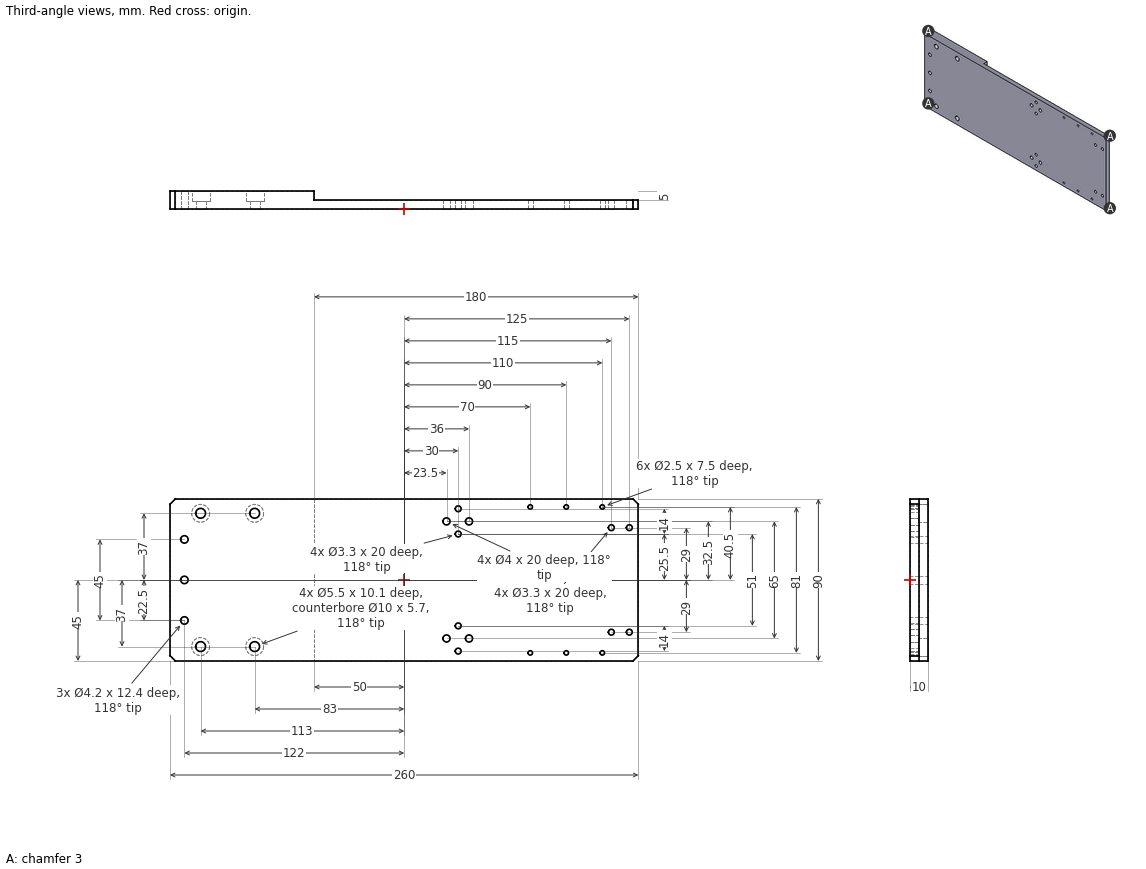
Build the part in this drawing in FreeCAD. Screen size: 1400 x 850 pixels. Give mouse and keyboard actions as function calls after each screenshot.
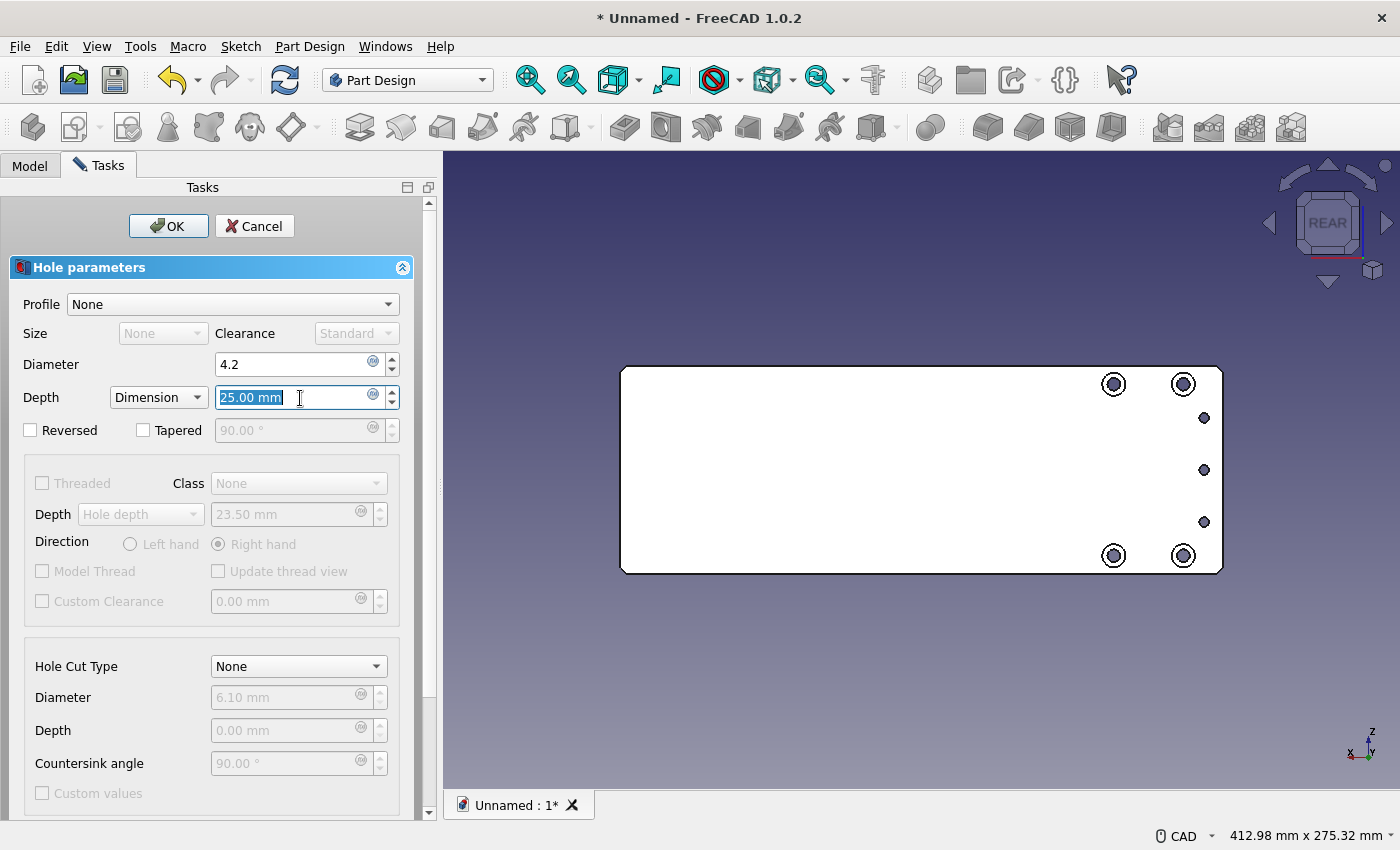
text(12.4)
key(Tab)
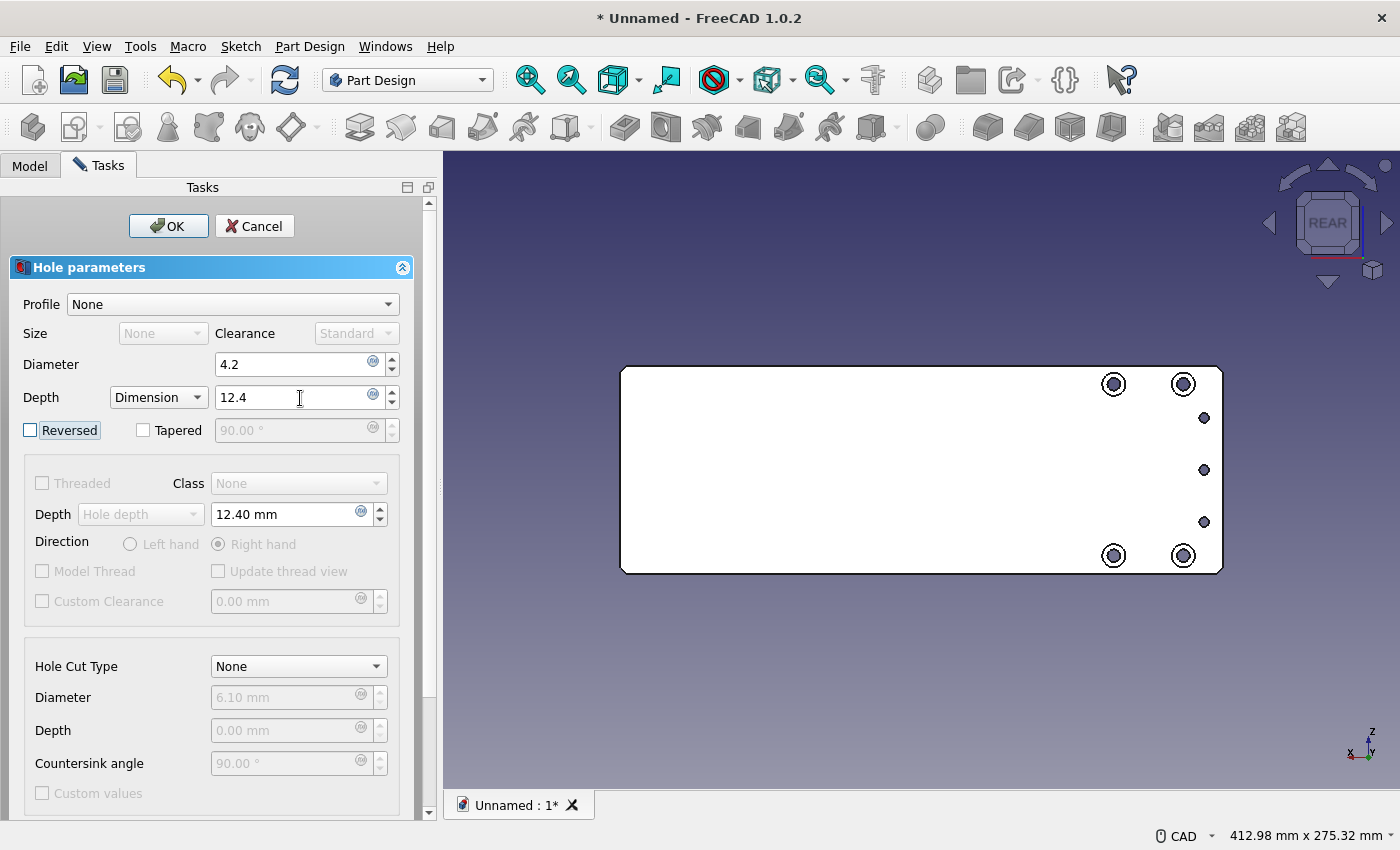
click(169, 226)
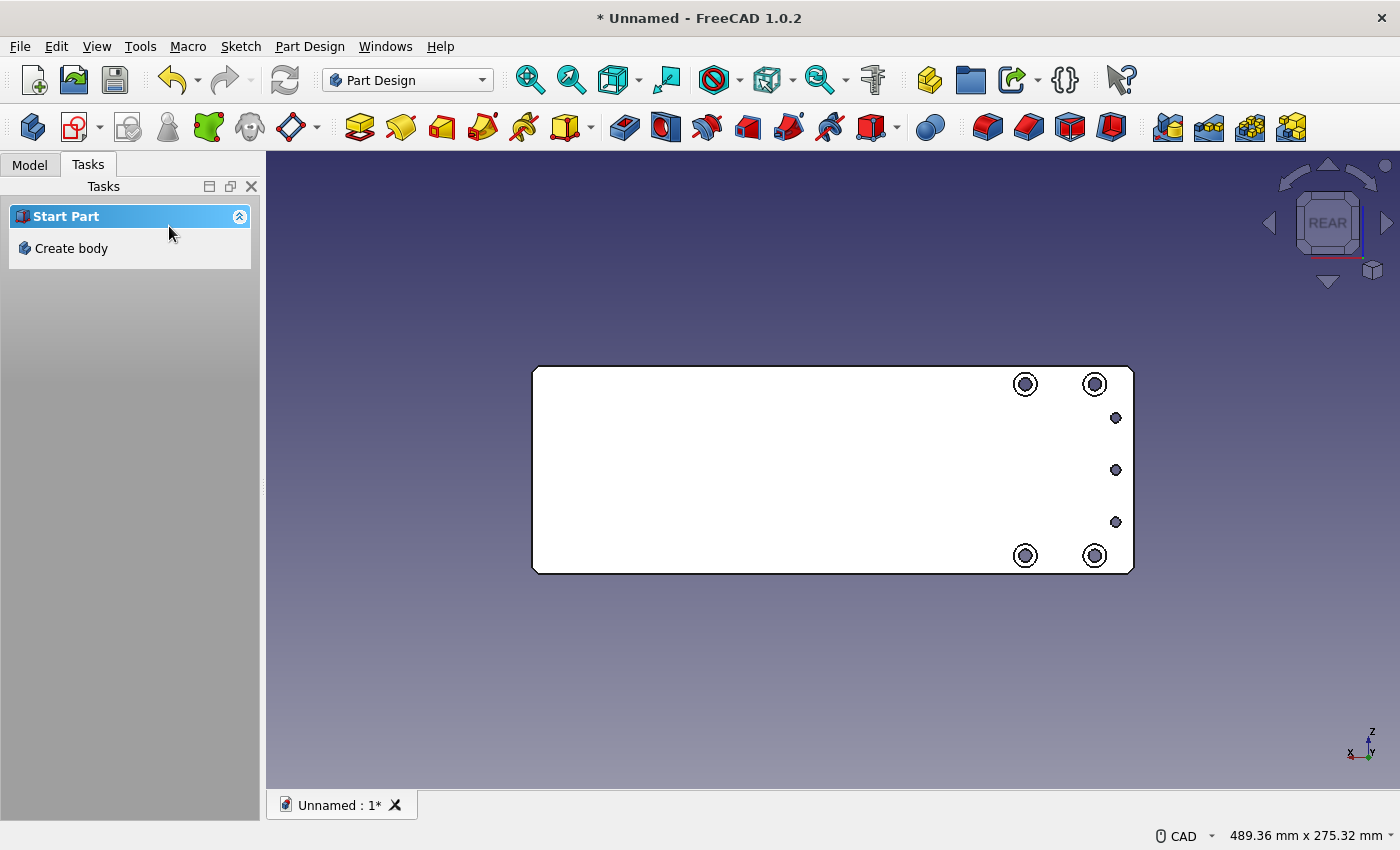
click(661, 469)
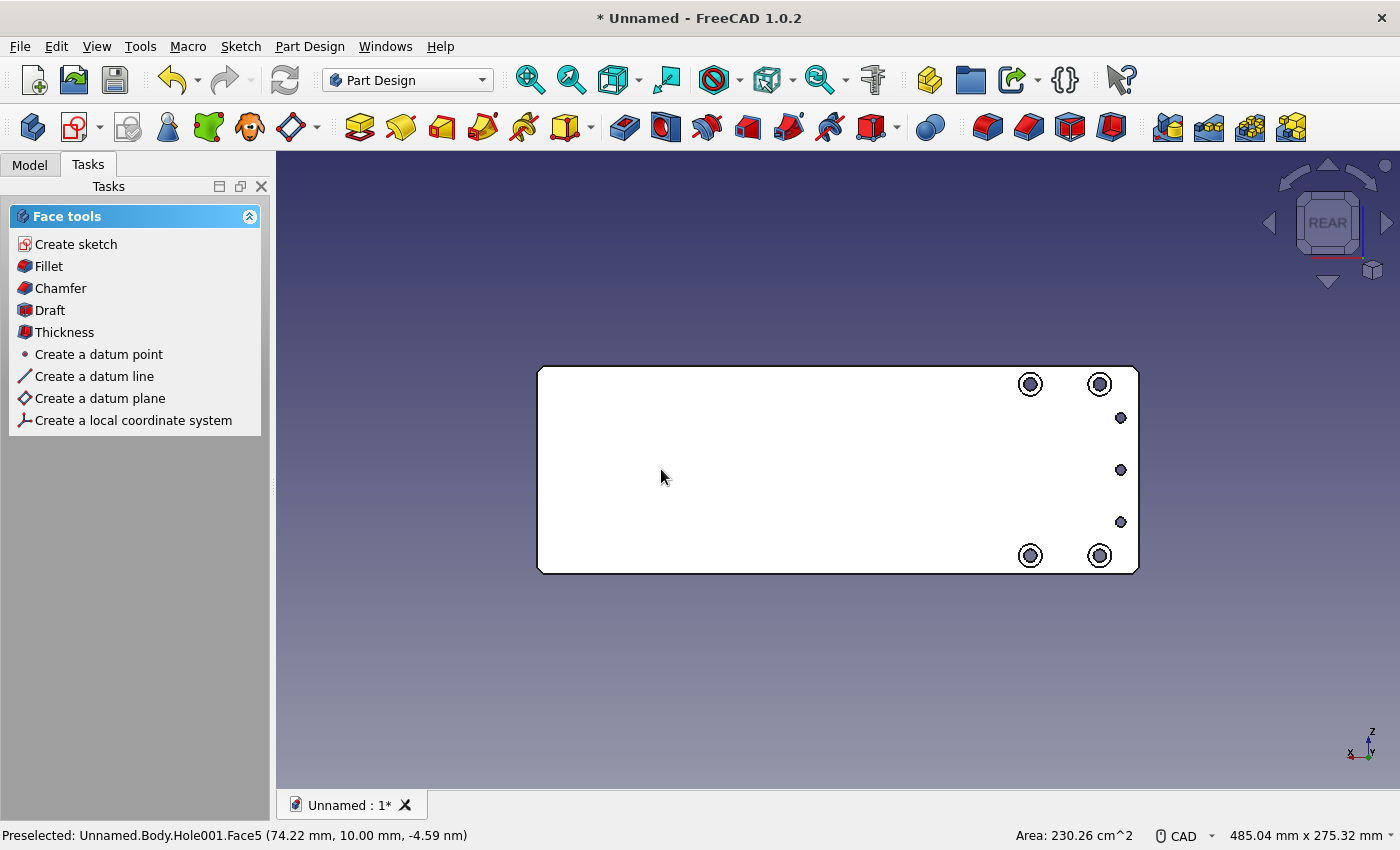
click(74, 128)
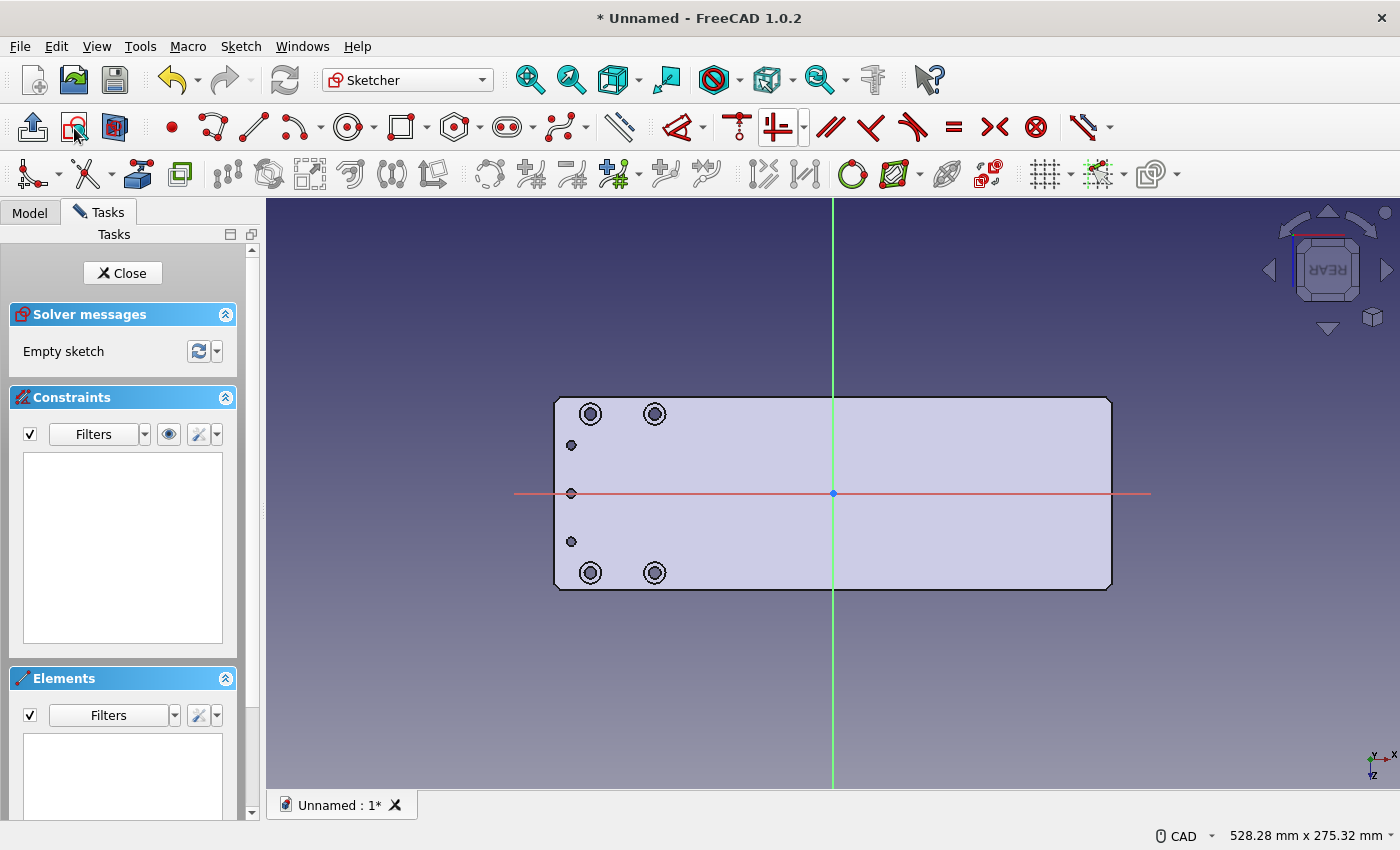
scroll(1107, 493, up, 3)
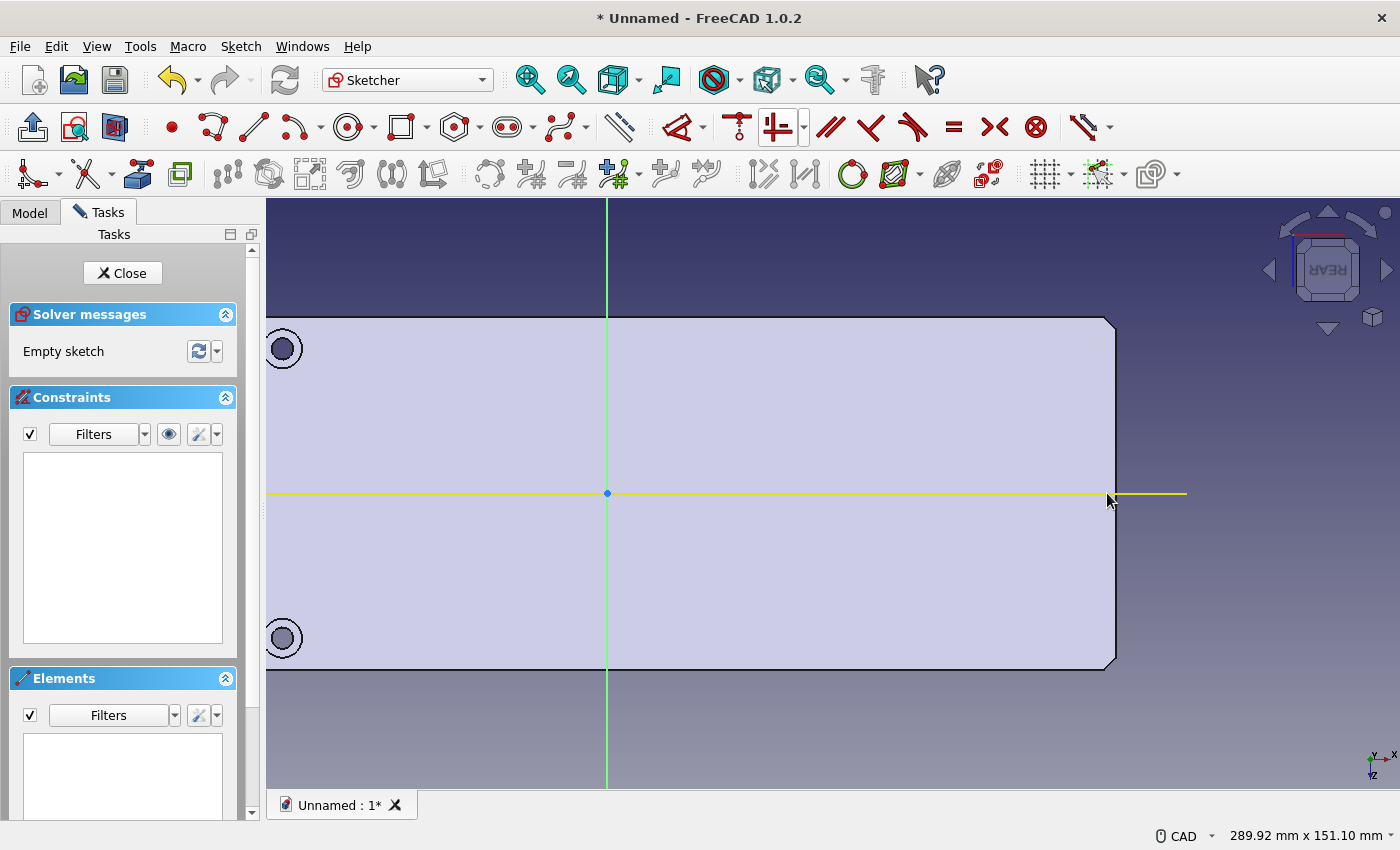
click(400, 128)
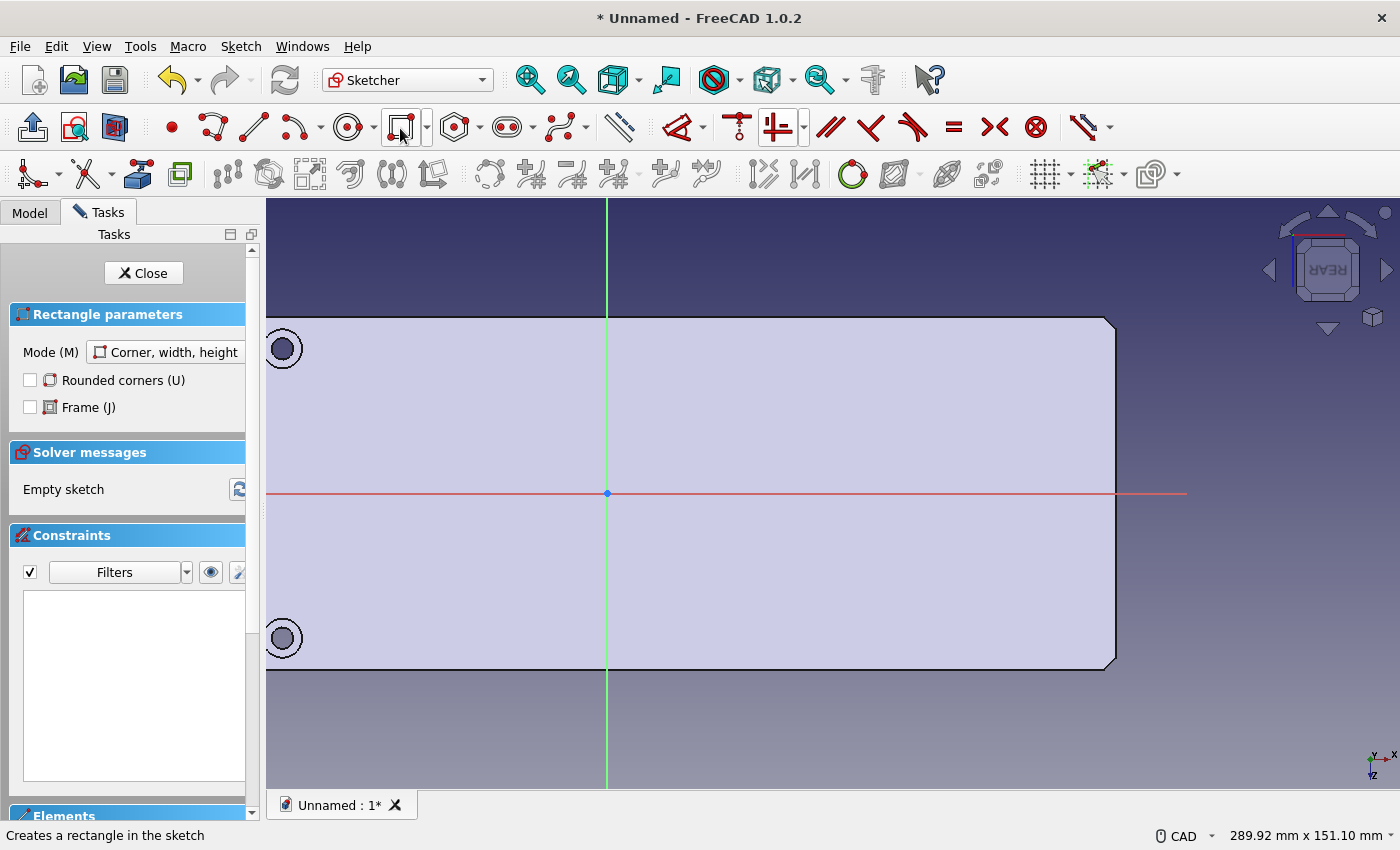
click(412, 317)
click(1116, 670)
key(Escape)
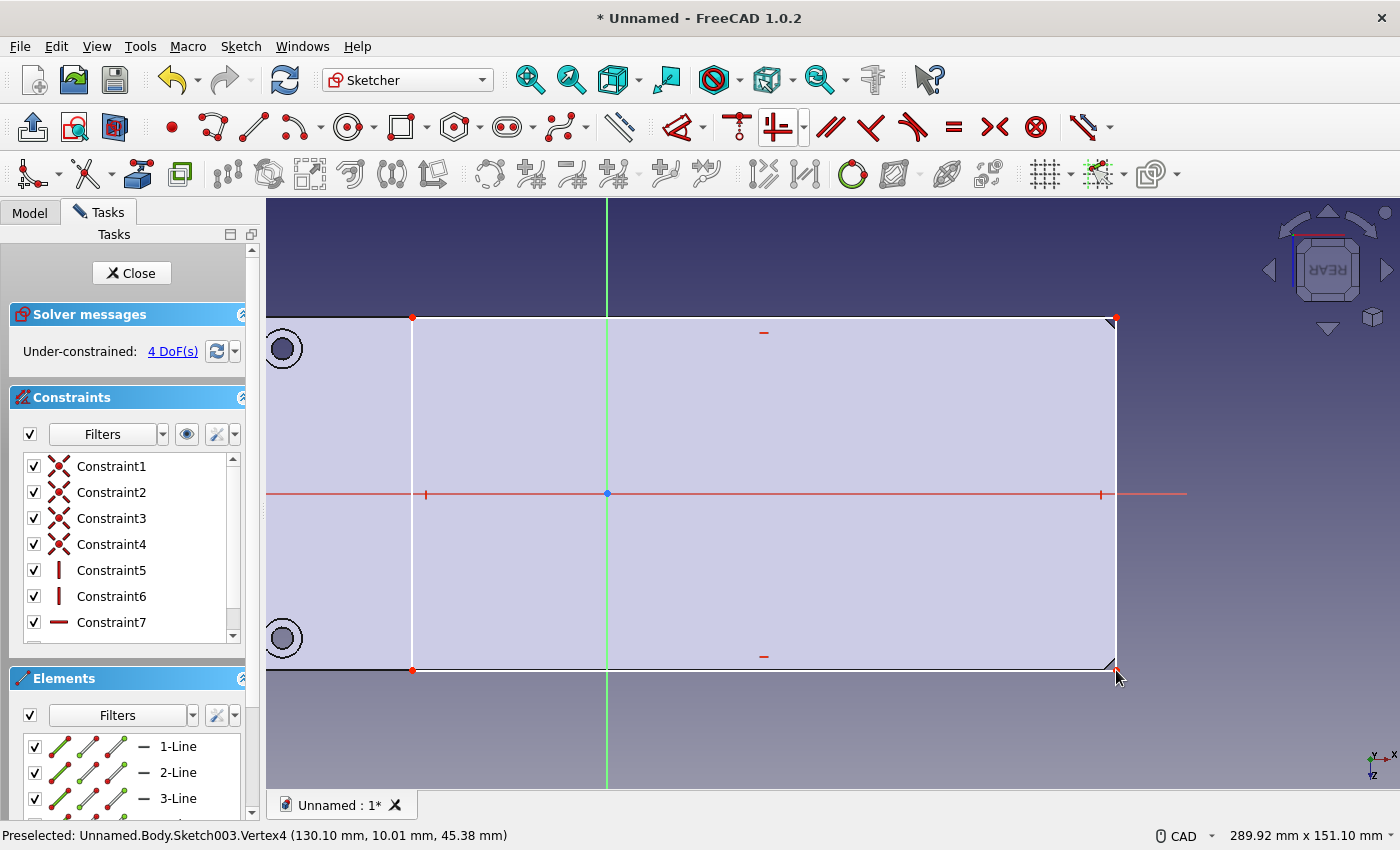
click(676, 128)